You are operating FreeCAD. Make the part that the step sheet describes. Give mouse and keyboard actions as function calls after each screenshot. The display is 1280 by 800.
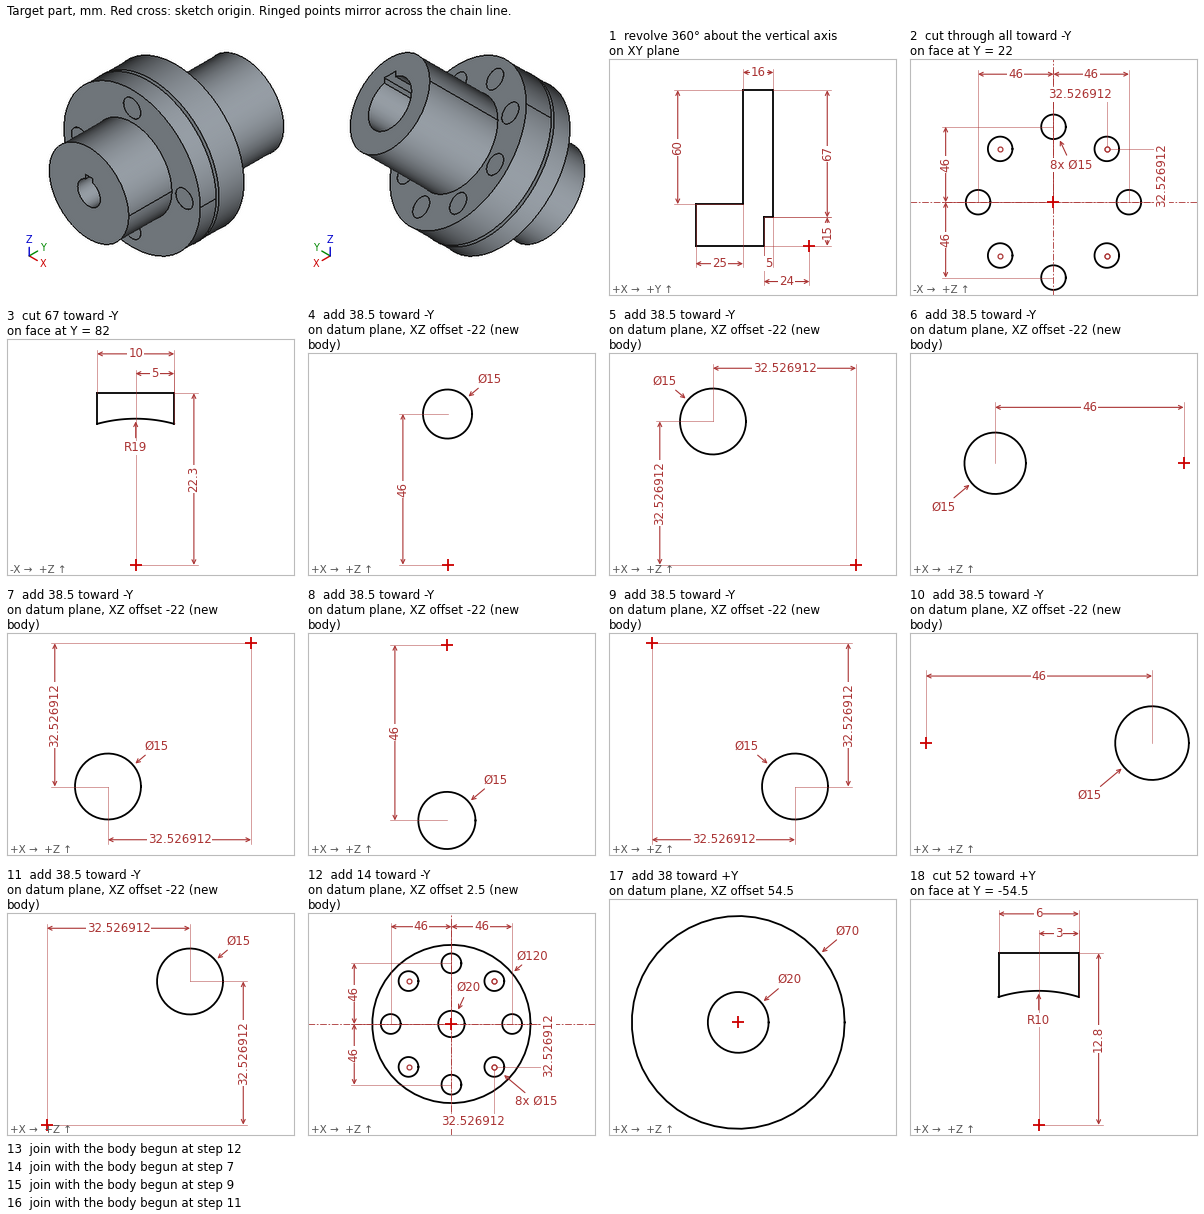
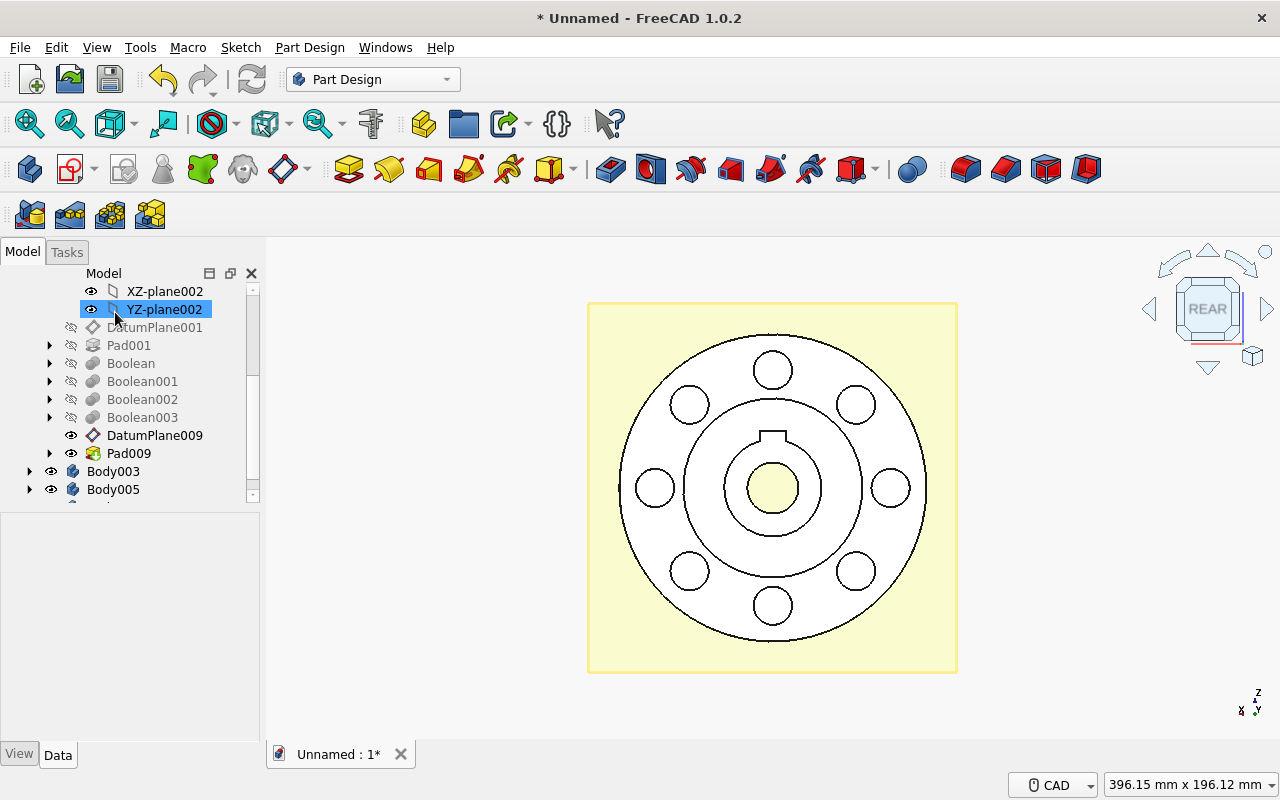
click(116, 435)
key(space)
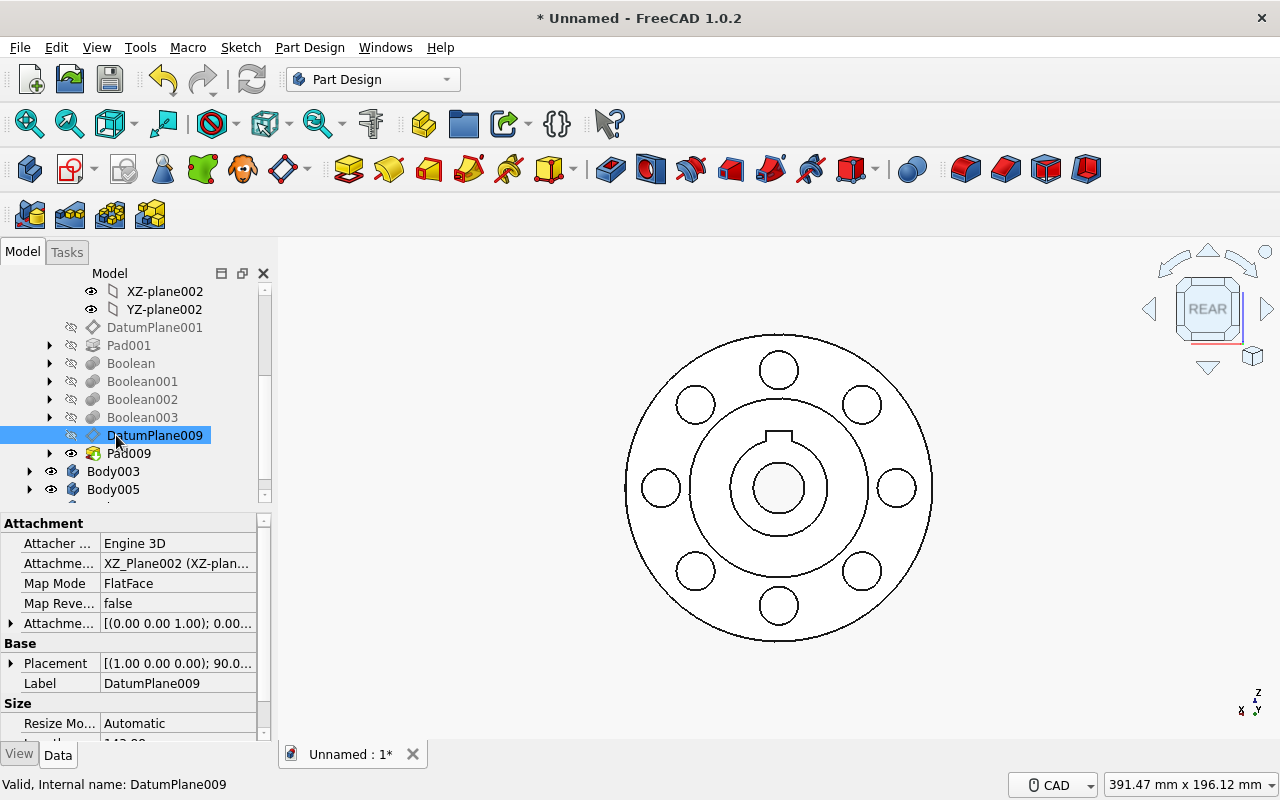
key(0)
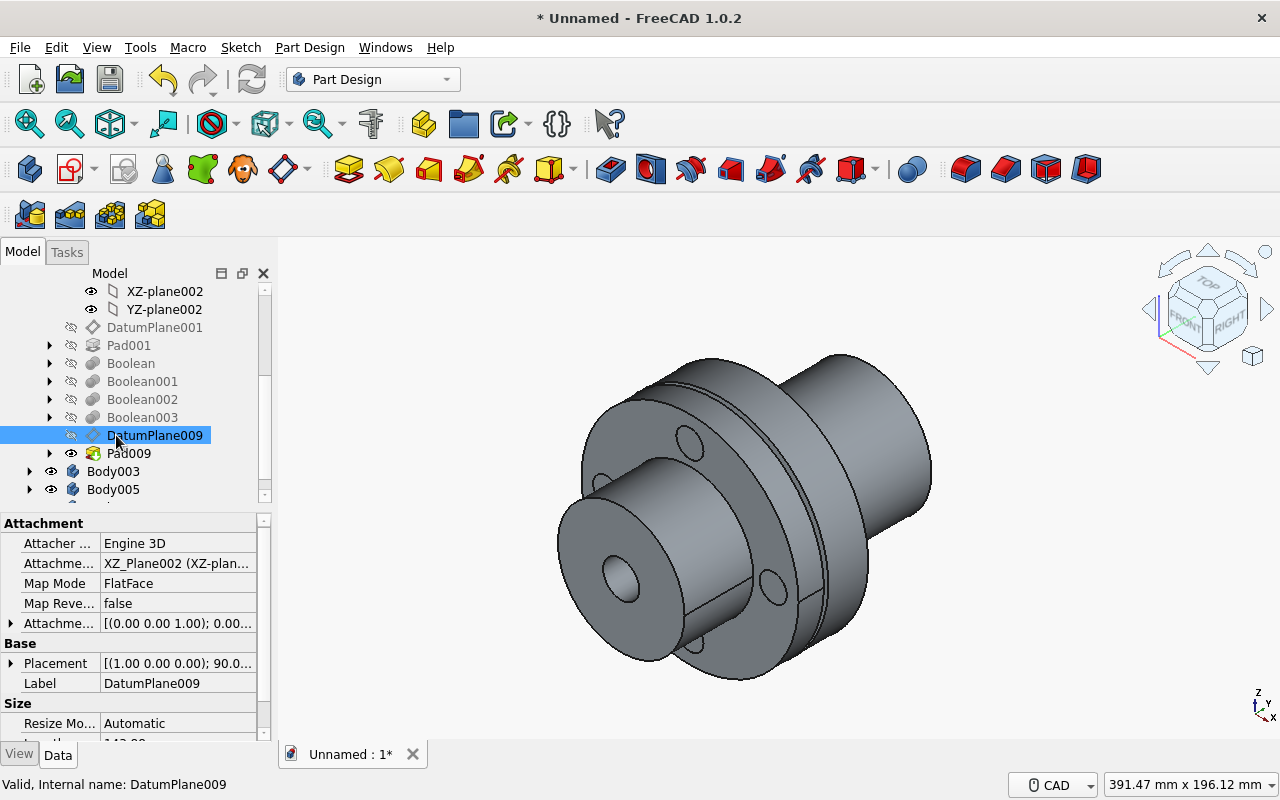
click(30, 124)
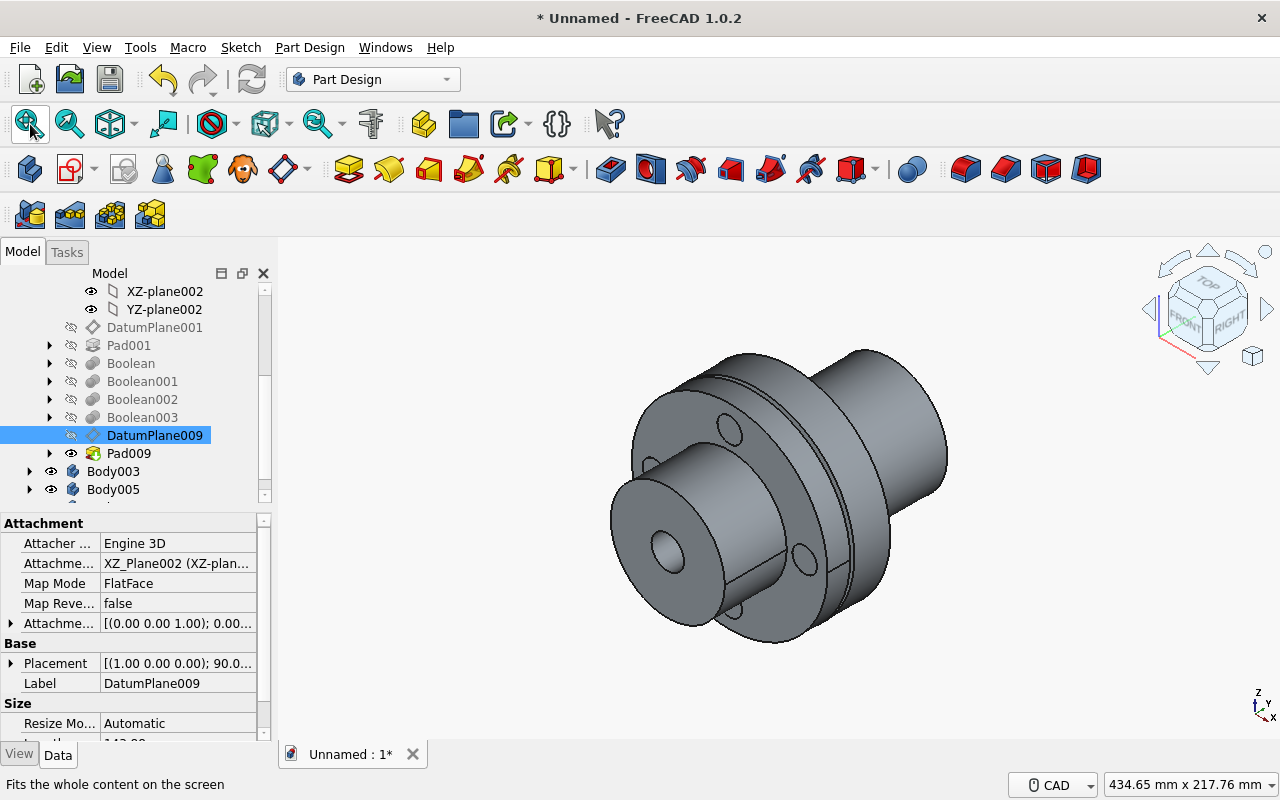
click(700, 551)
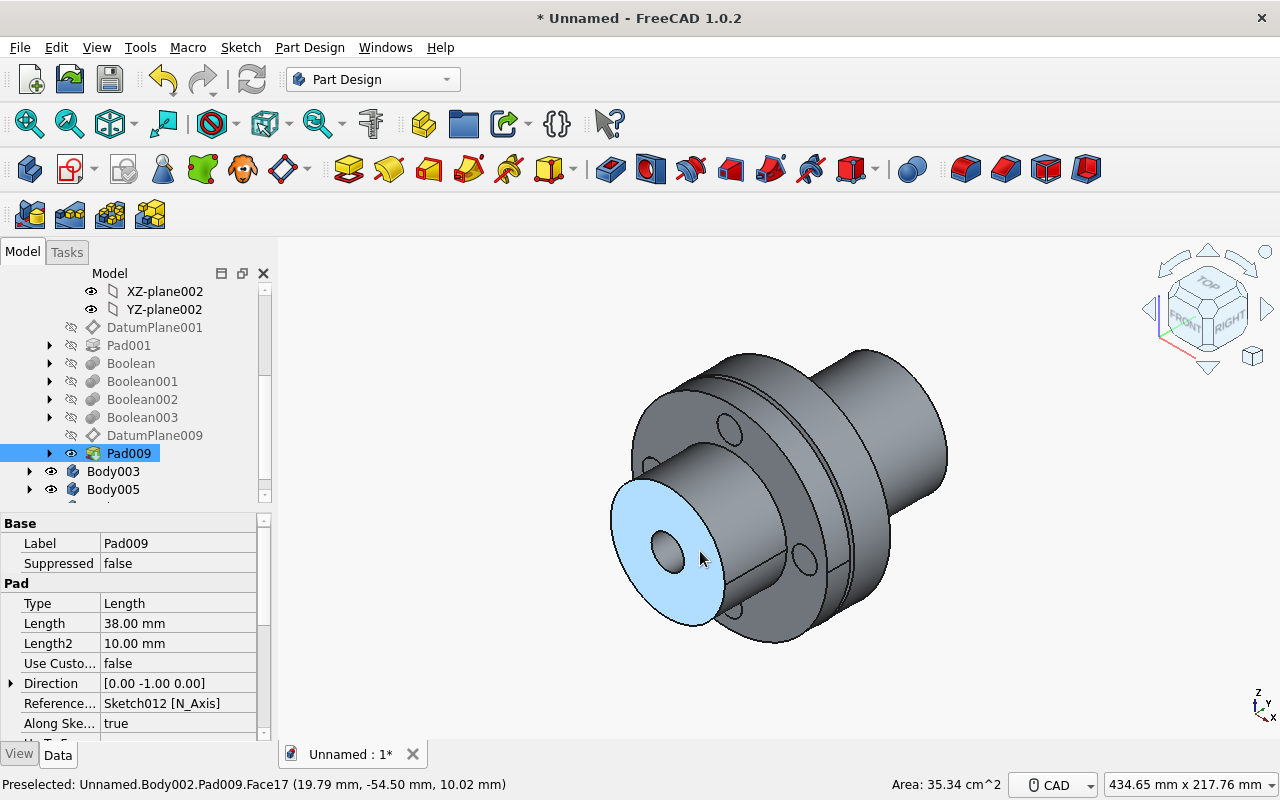
click(70, 170)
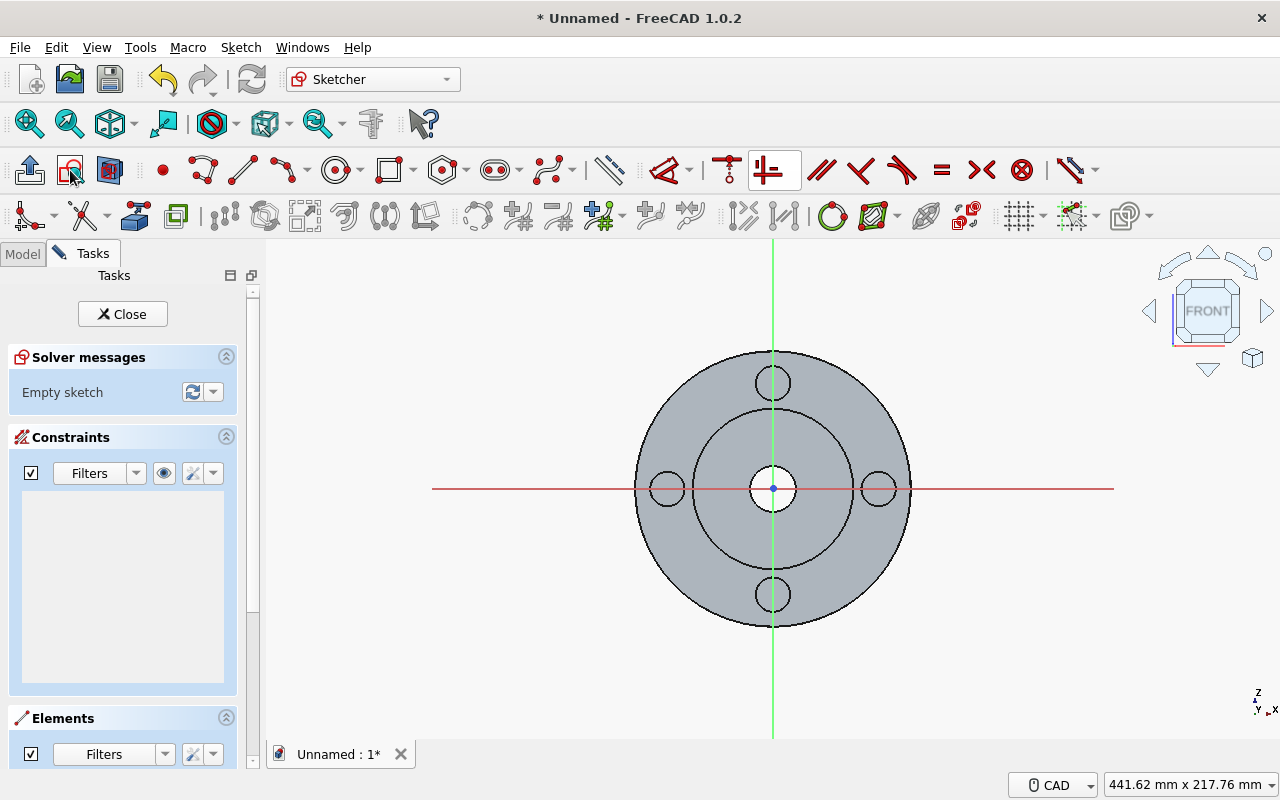
scroll(780, 473, up, 12)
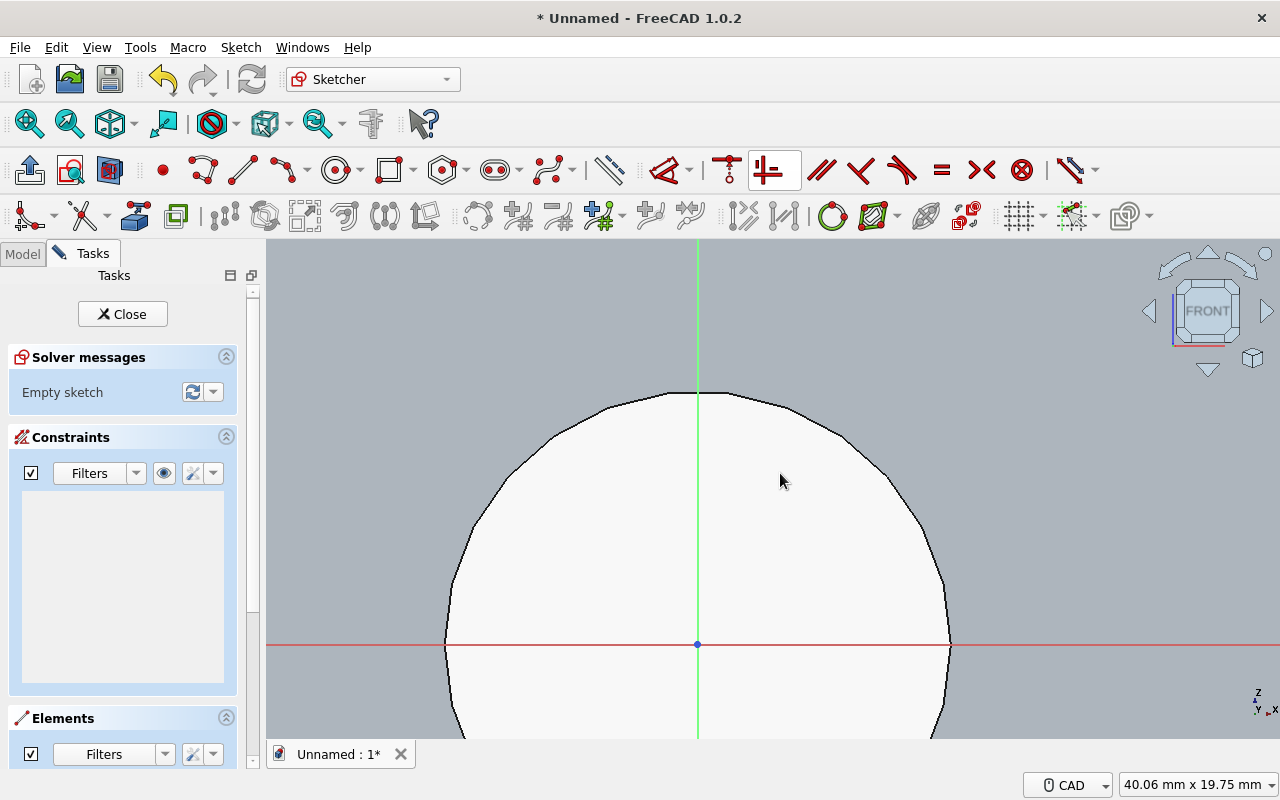
click(204, 170)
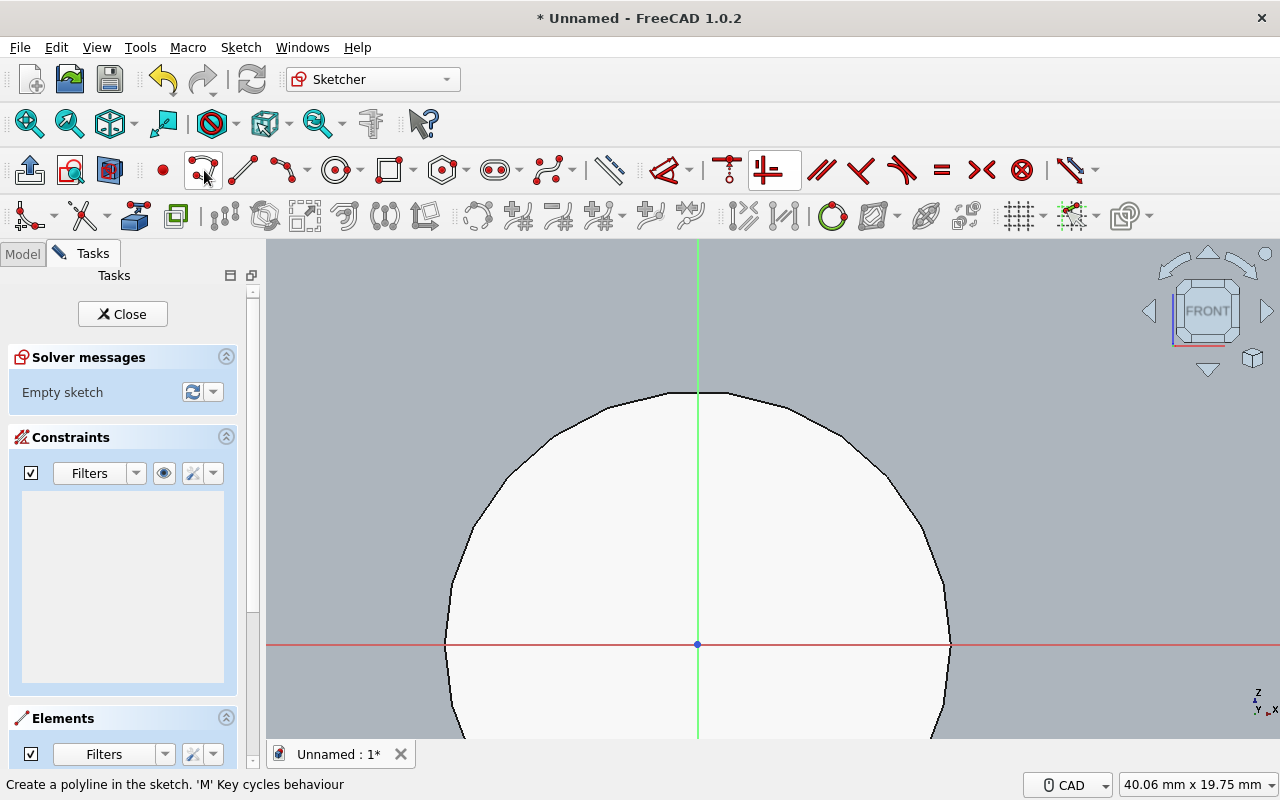
click(774, 403)
click(774, 321)
click(622, 321)
click(622, 403)
right_click(622, 403)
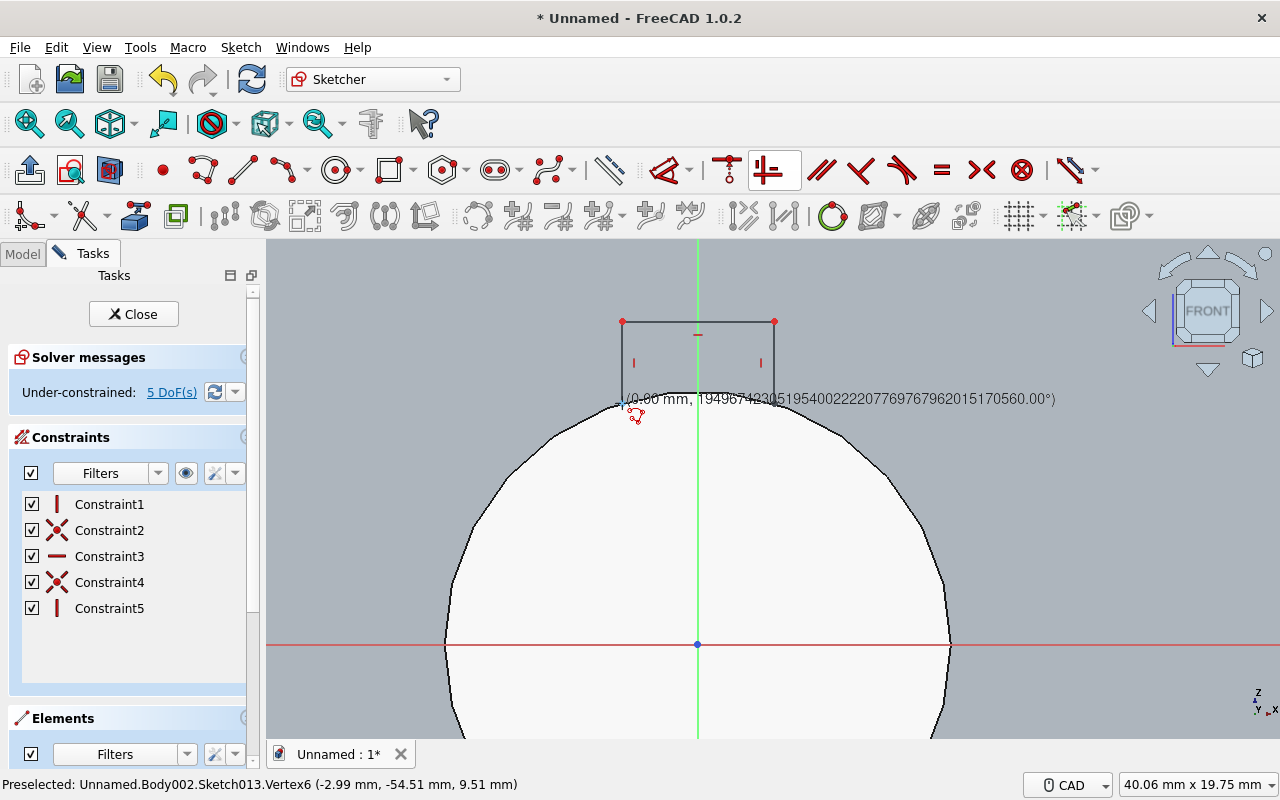
click(284, 170)